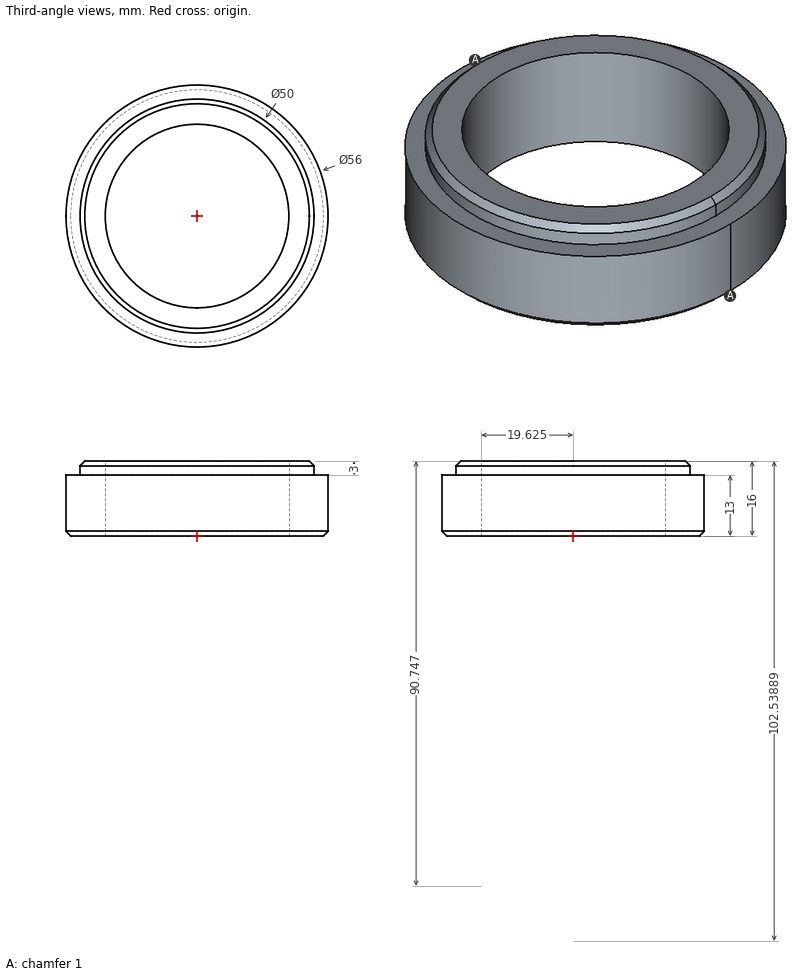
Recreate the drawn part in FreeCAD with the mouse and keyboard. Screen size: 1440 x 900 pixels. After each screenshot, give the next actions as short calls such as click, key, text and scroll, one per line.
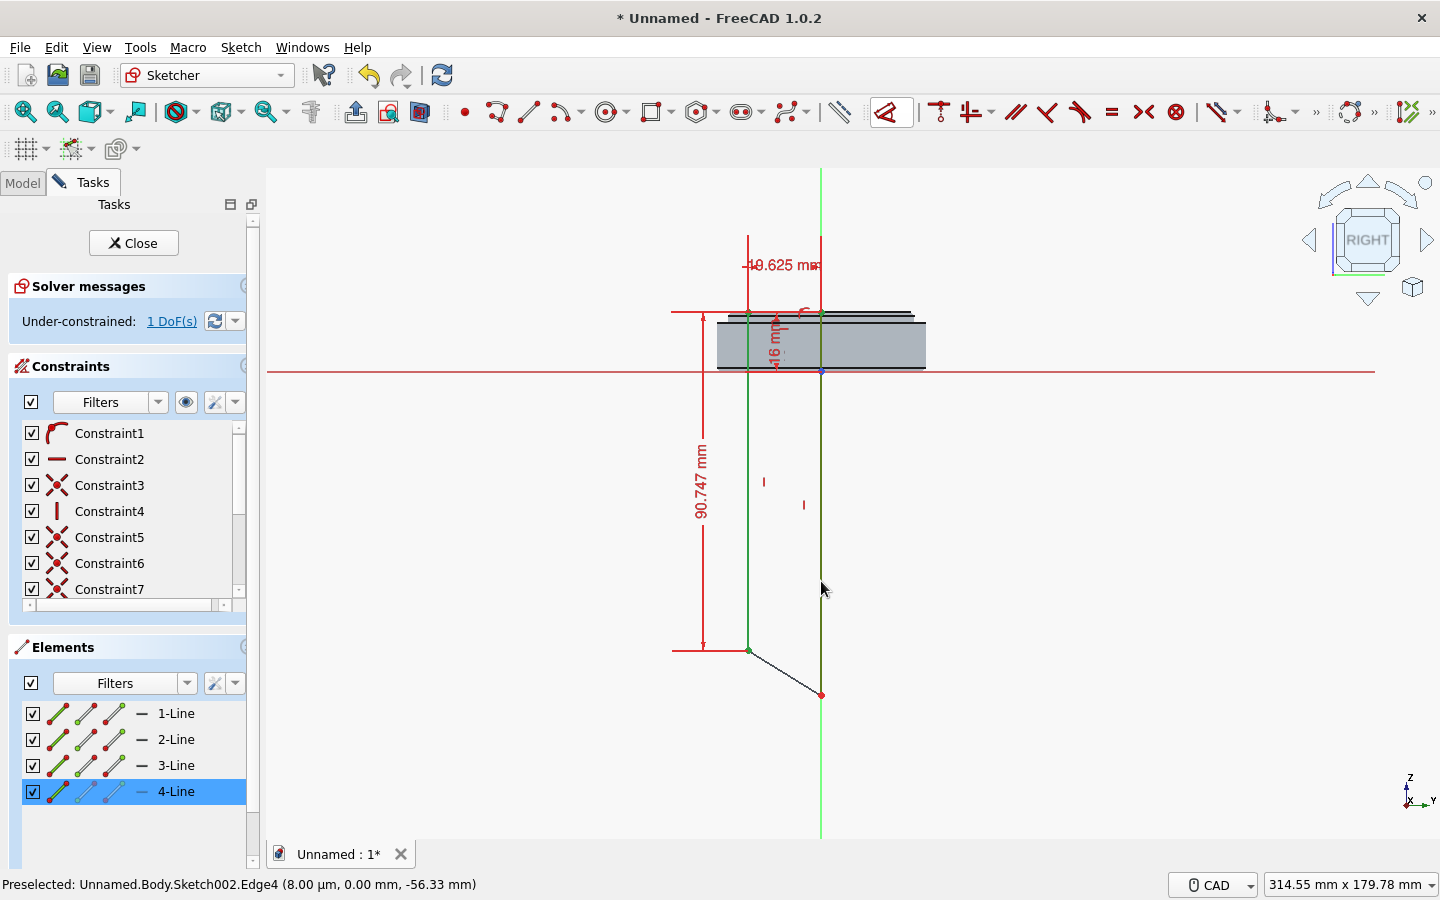
click(908, 112)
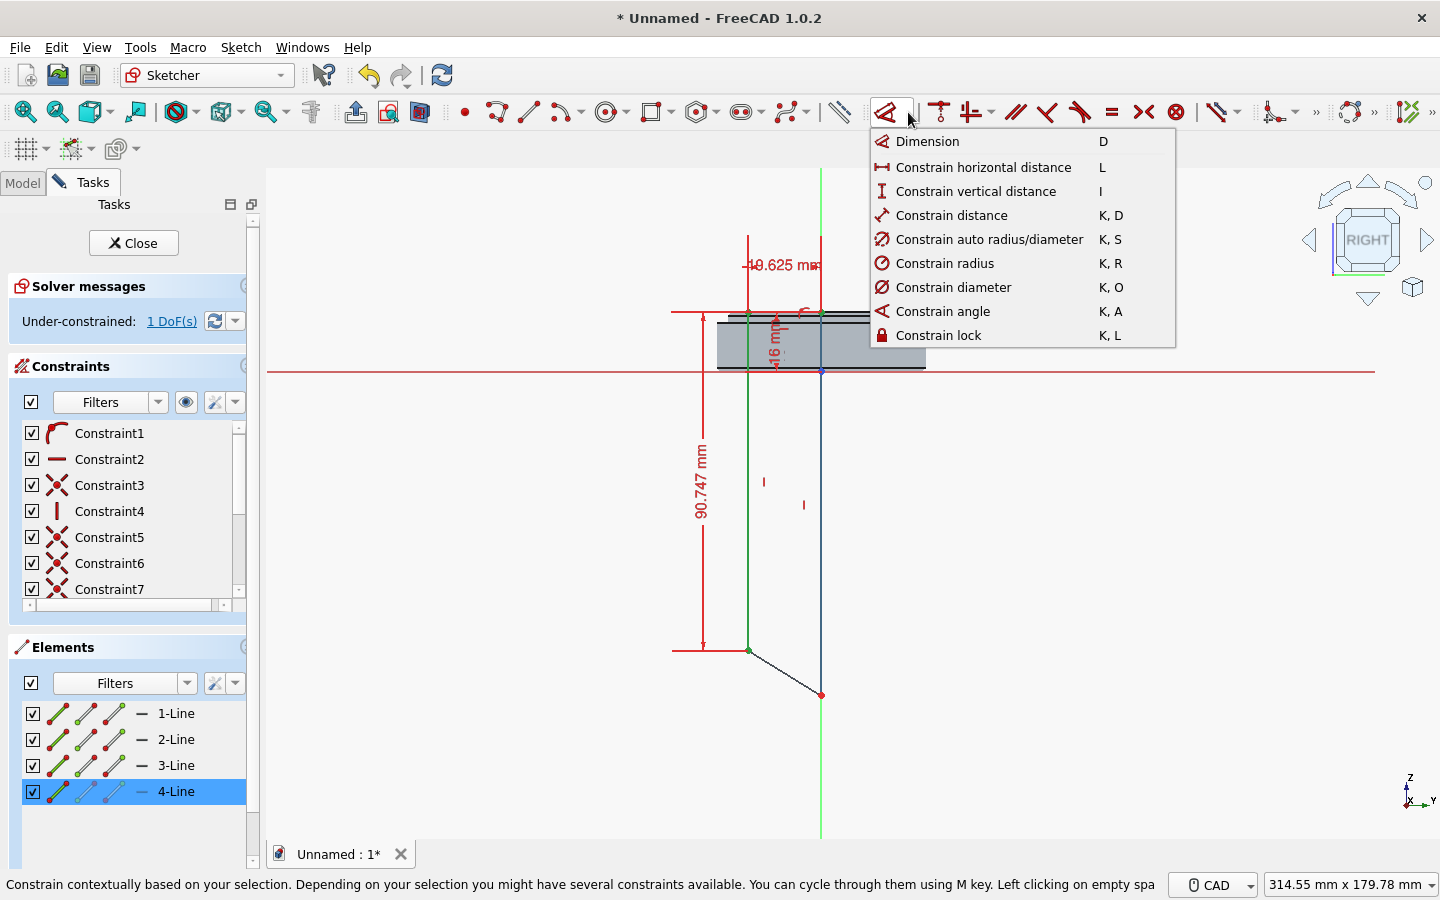
click(1023, 191)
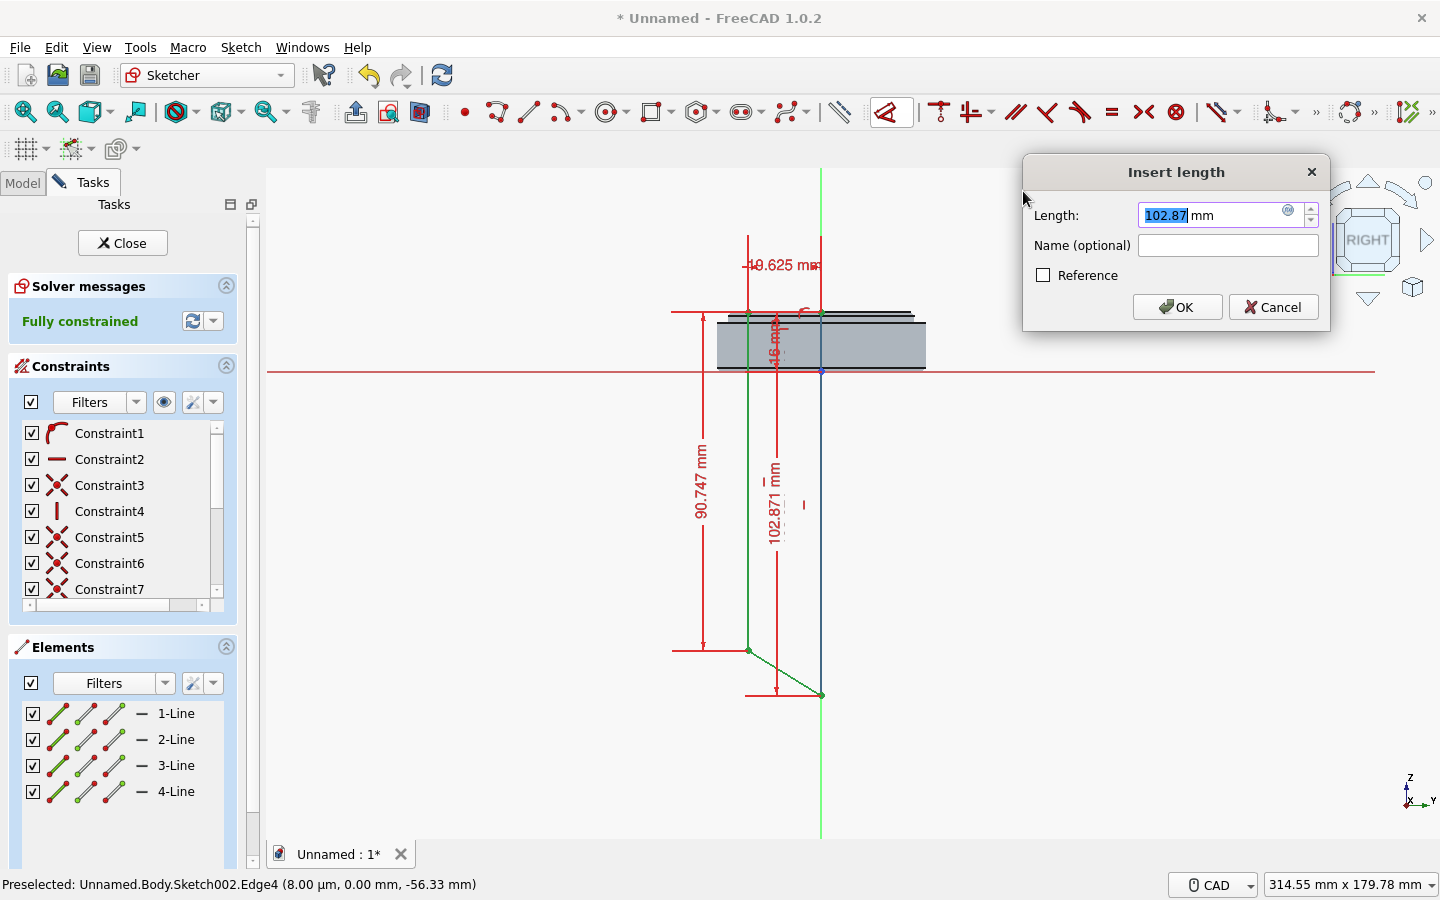
text(102.53889)
key(Return)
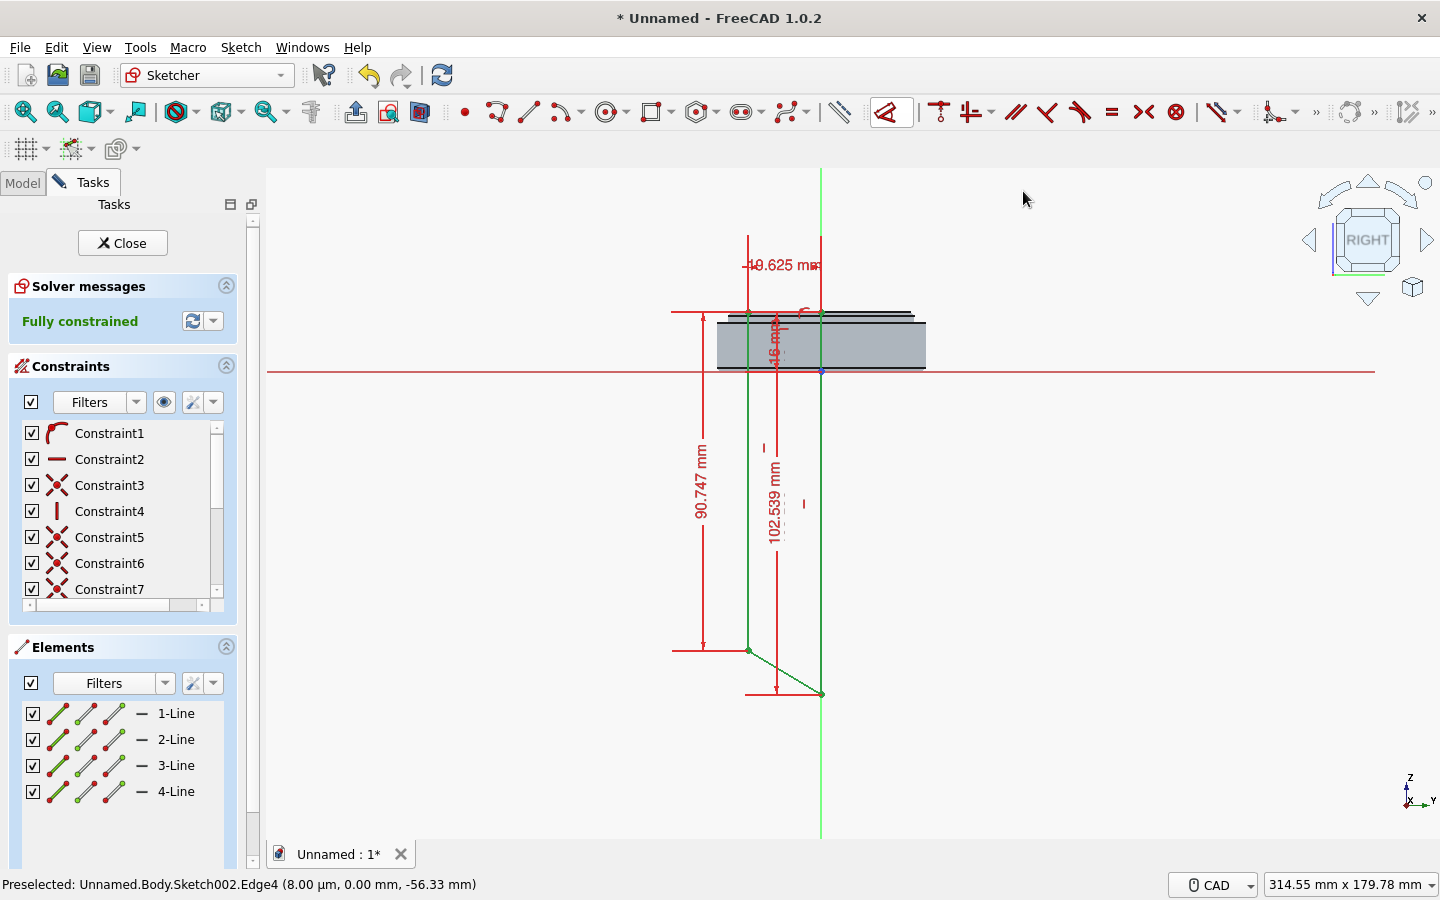
click(123, 243)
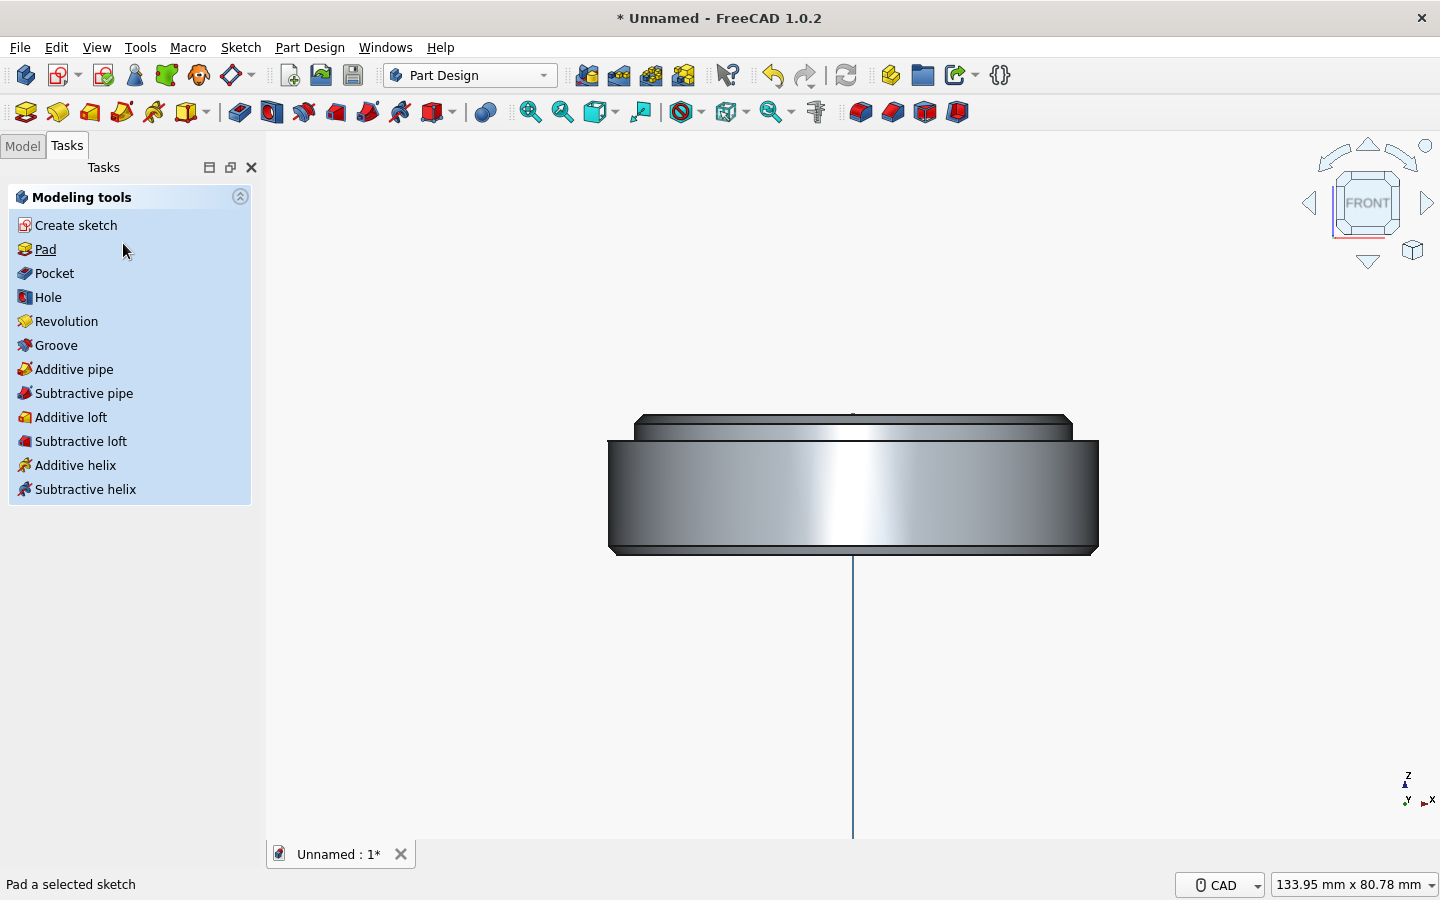
click(304, 112)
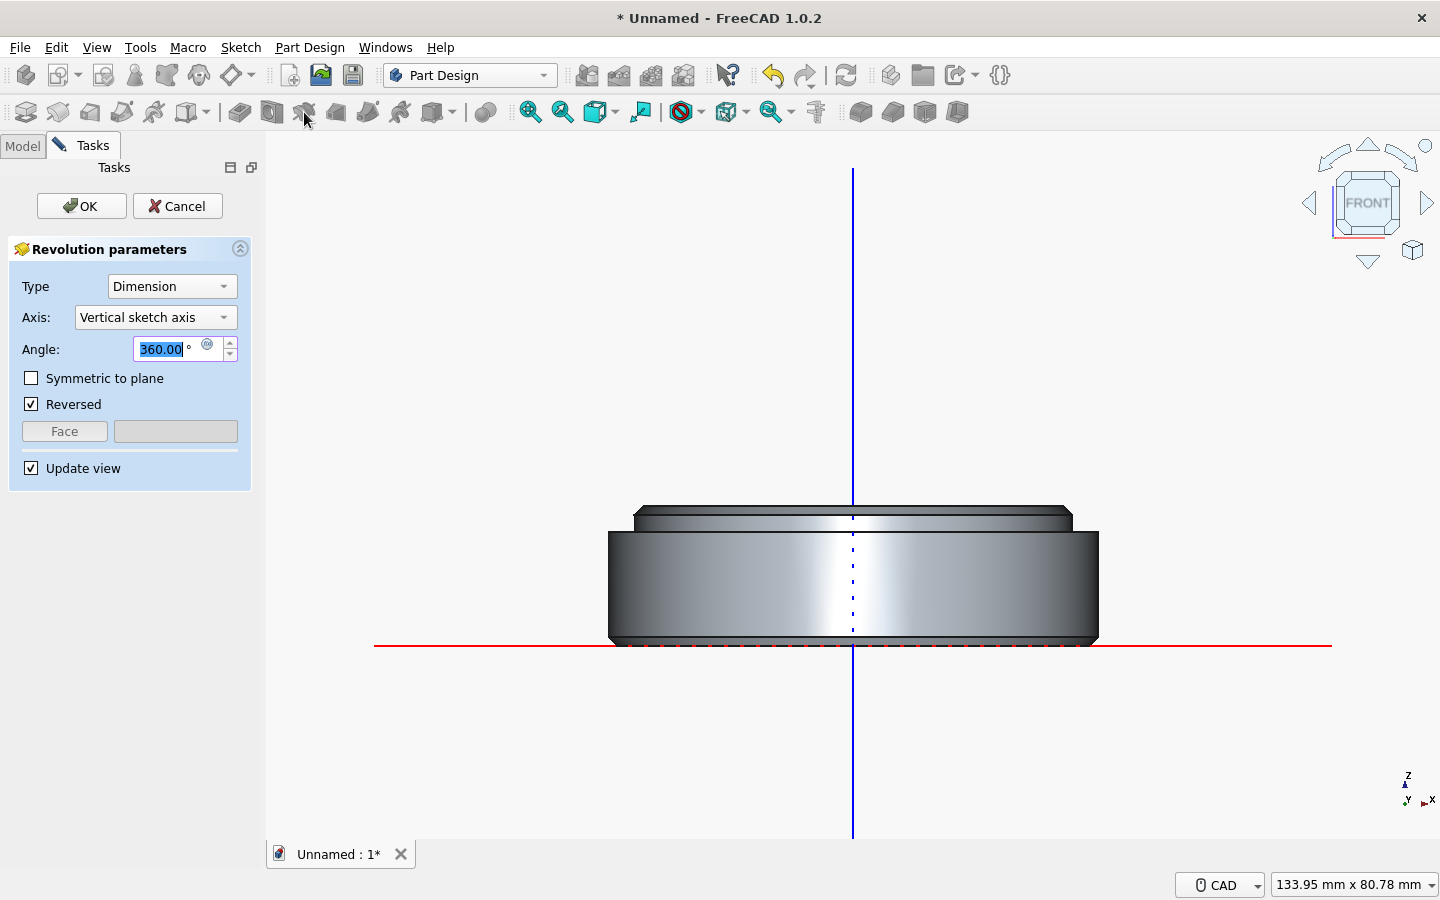
click(82, 206)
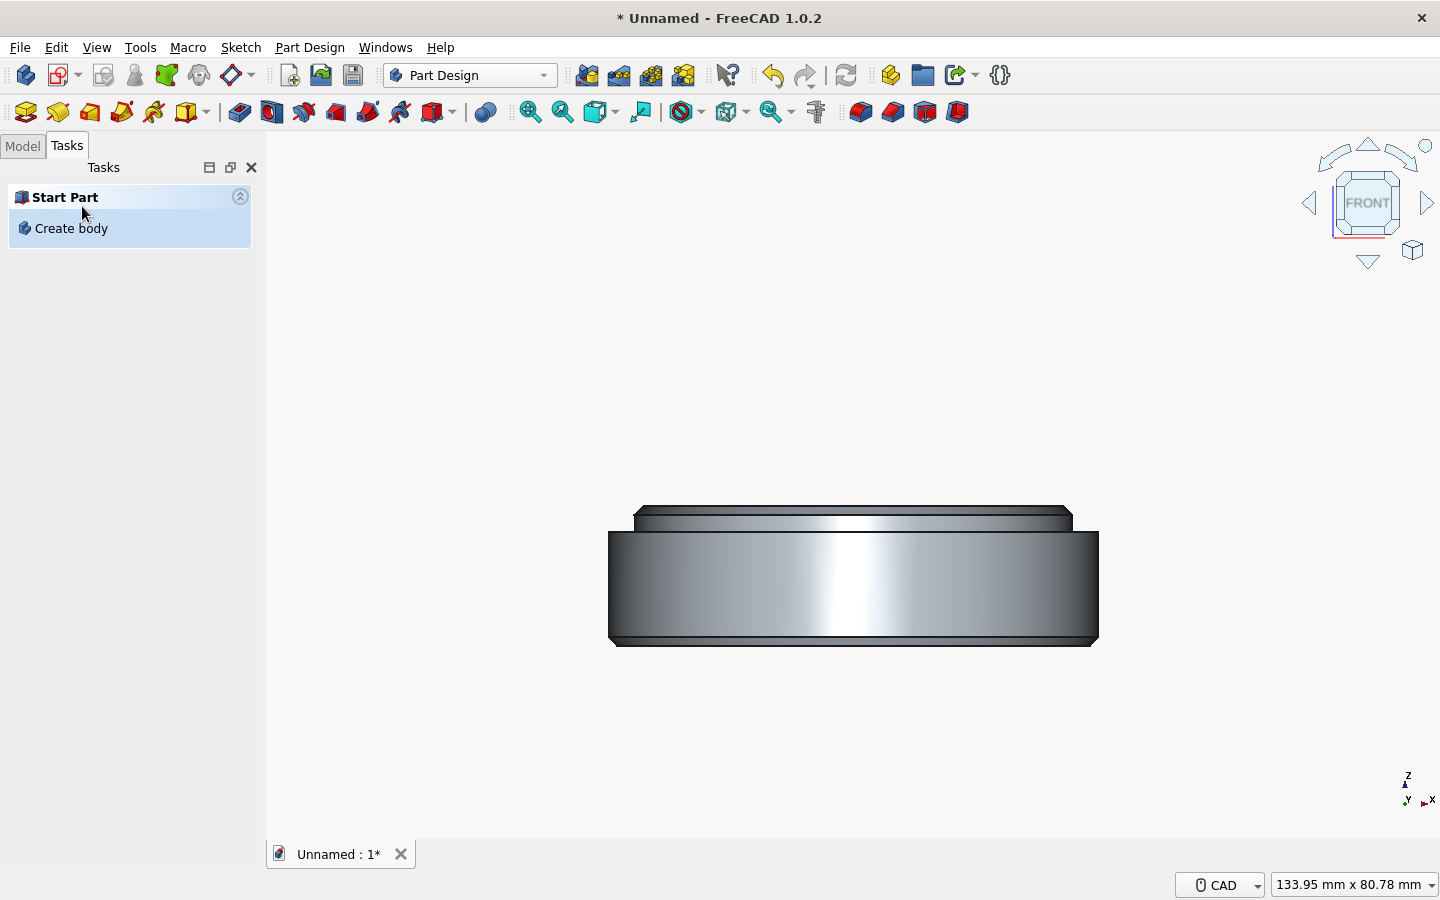
key(0)